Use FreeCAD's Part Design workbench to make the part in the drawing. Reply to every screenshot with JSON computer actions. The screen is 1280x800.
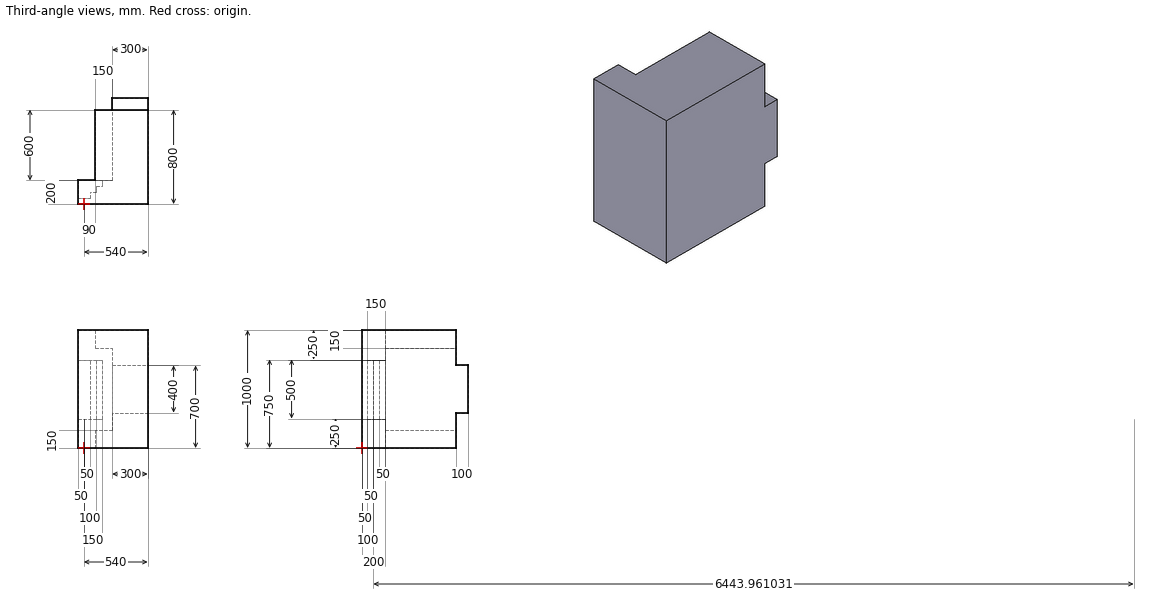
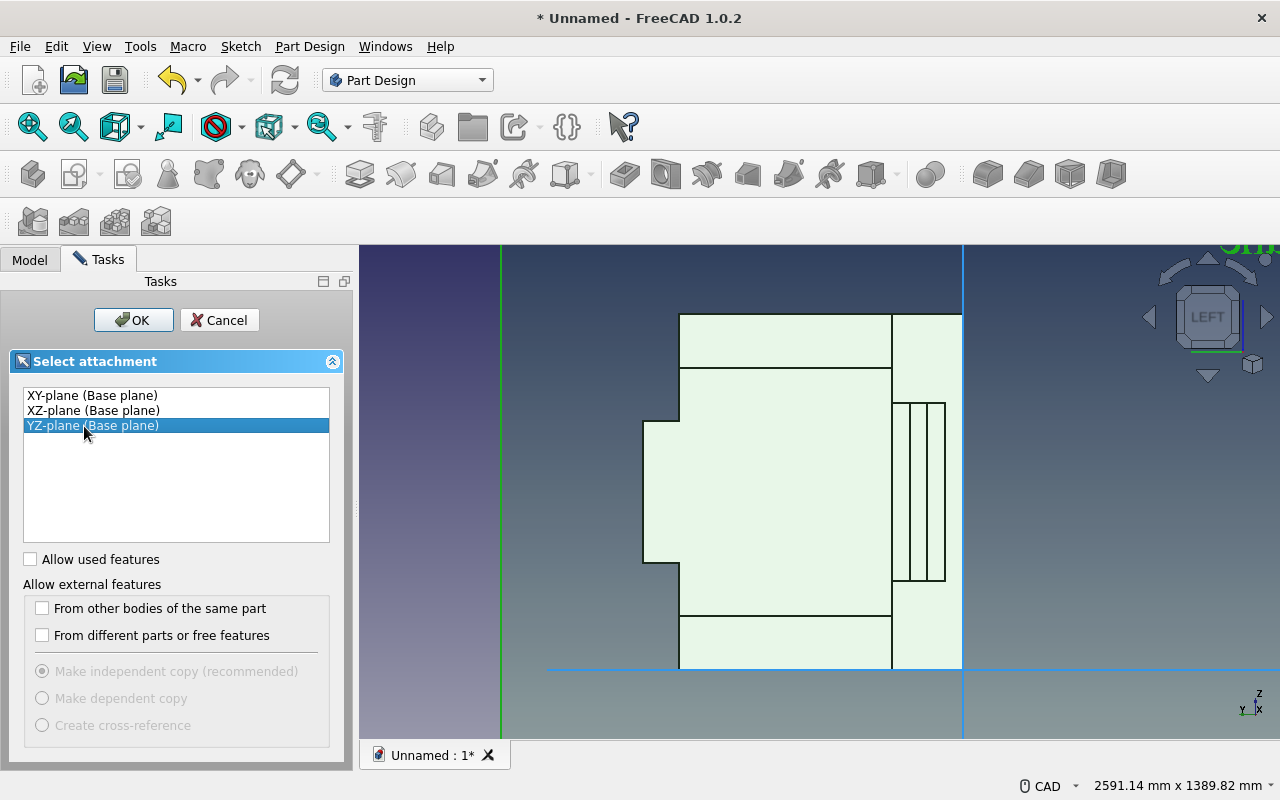
{"action": "left_click", "coordinate": [134, 320]}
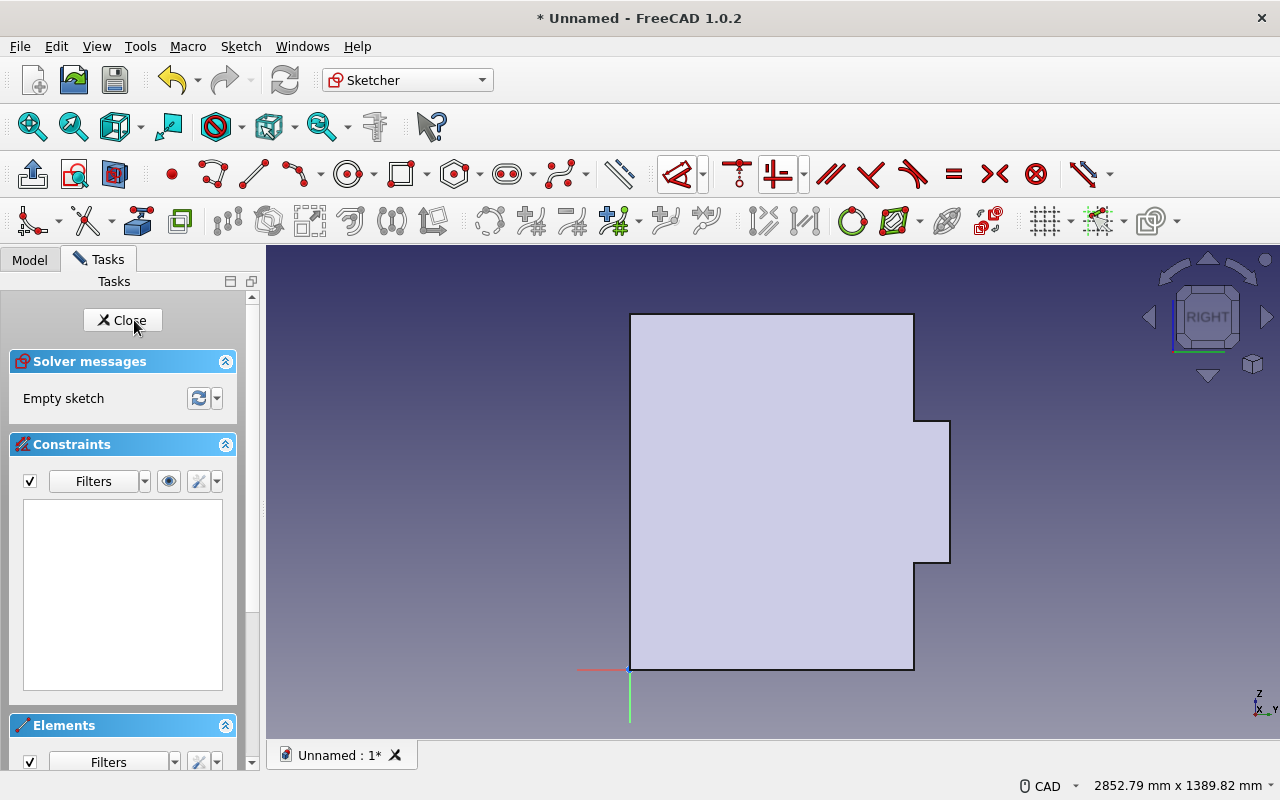
{"action": "left_click", "coordinate": [115, 174]}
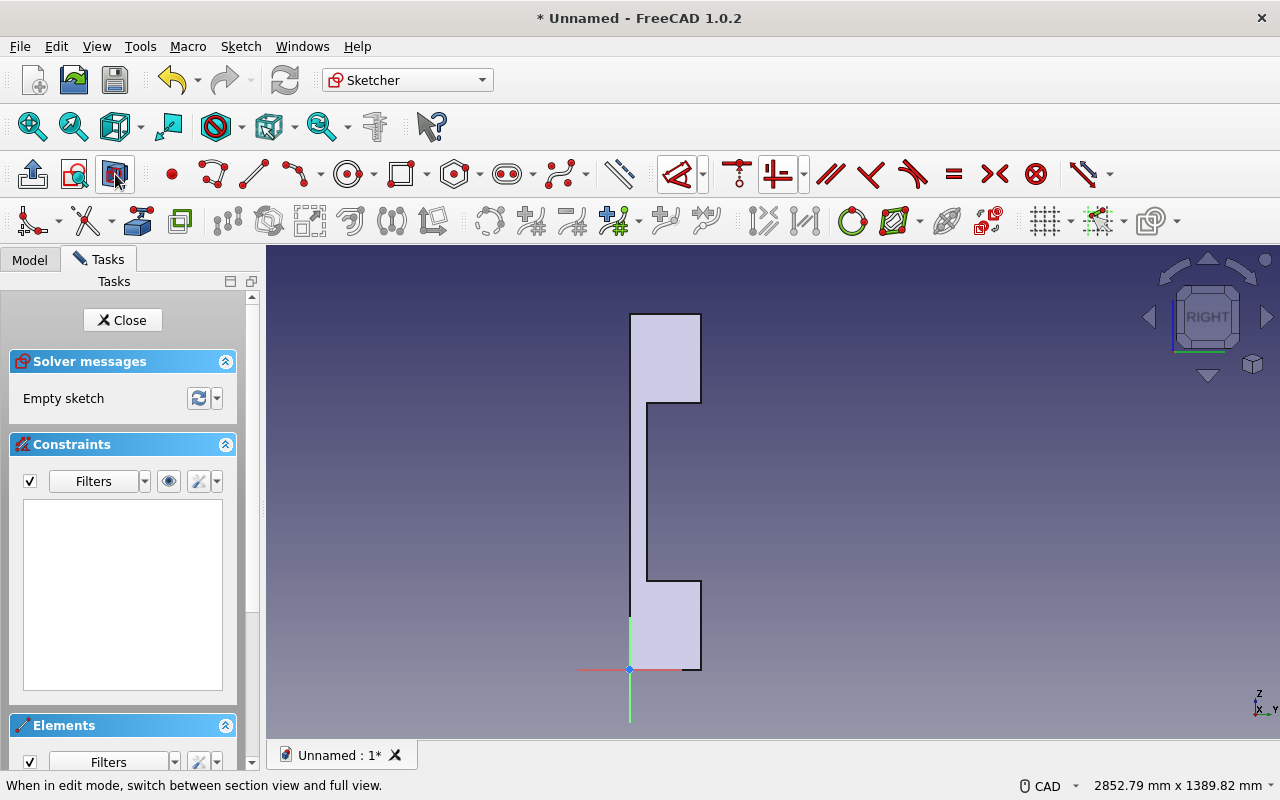
{"action": "left_click", "coordinate": [213, 174]}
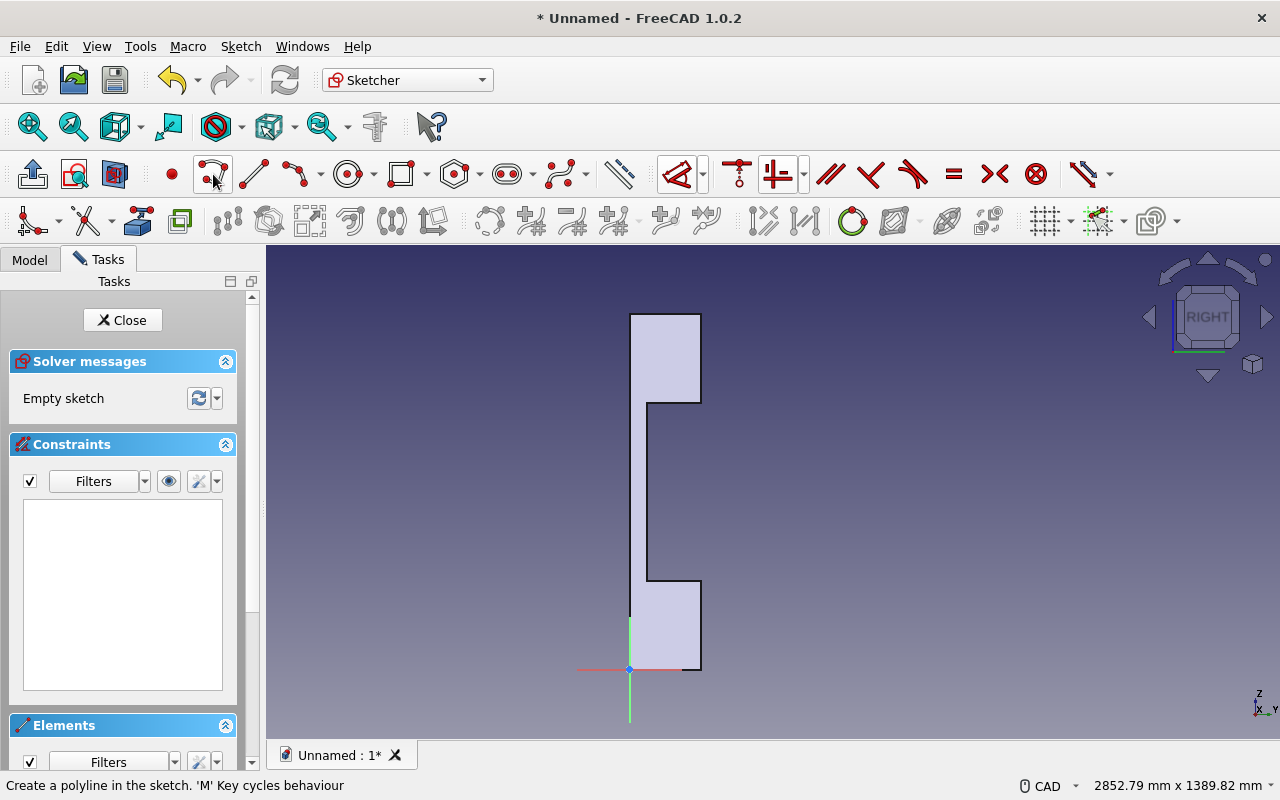
{"action": "left_click", "coordinate": [630, 670]}
{"action": "left_click", "coordinate": [639, 314]}
{"action": "left_click", "coordinate": [701, 314]}
{"action": "left_click", "coordinate": [701, 403]}
{"action": "left_click", "coordinate": [647, 403]}
{"action": "left_click", "coordinate": [647, 581]}
{"action": "left_click", "coordinate": [701, 581]}
{"action": "left_click", "coordinate": [701, 661]}
{"action": "left_click", "coordinate": [630, 670]}
{"action": "key", "text": "Escape"}
{"action": "key", "text": "Escape"}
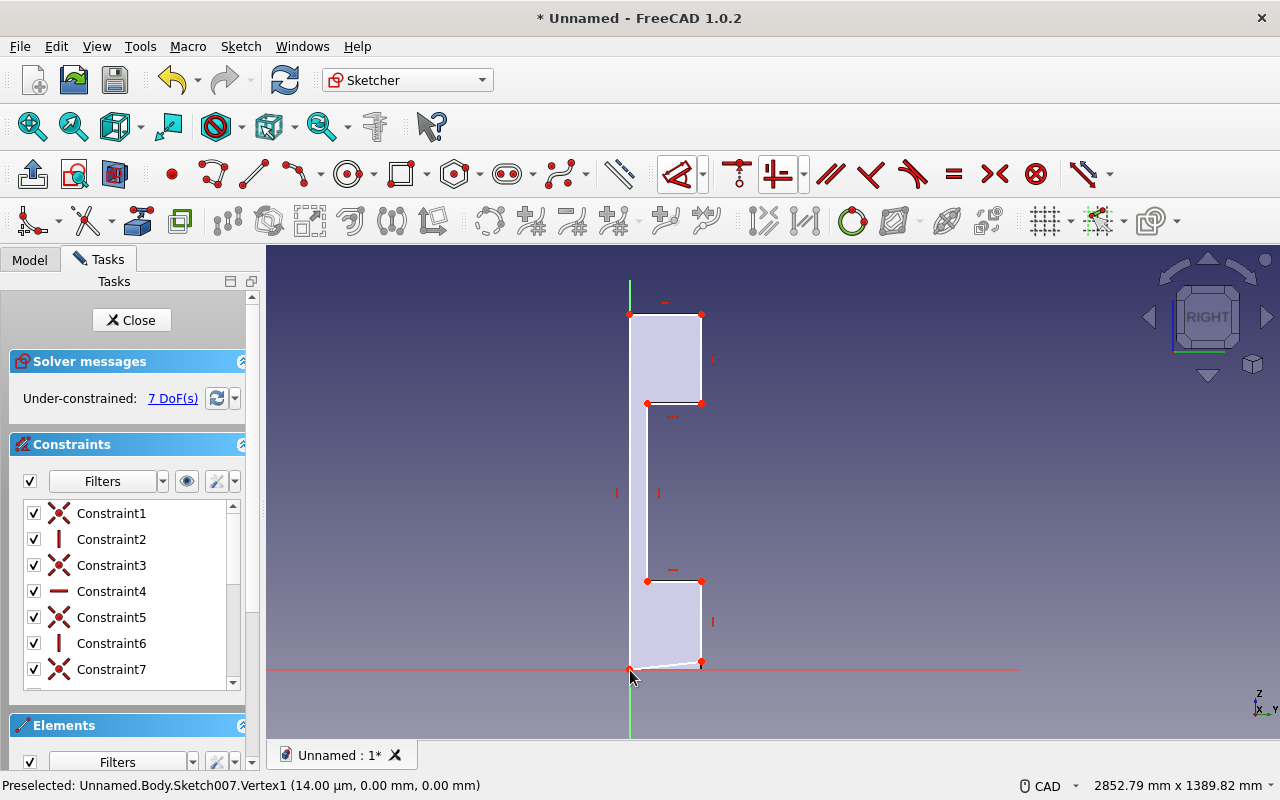
{"action": "left_click", "coordinate": [651, 667]}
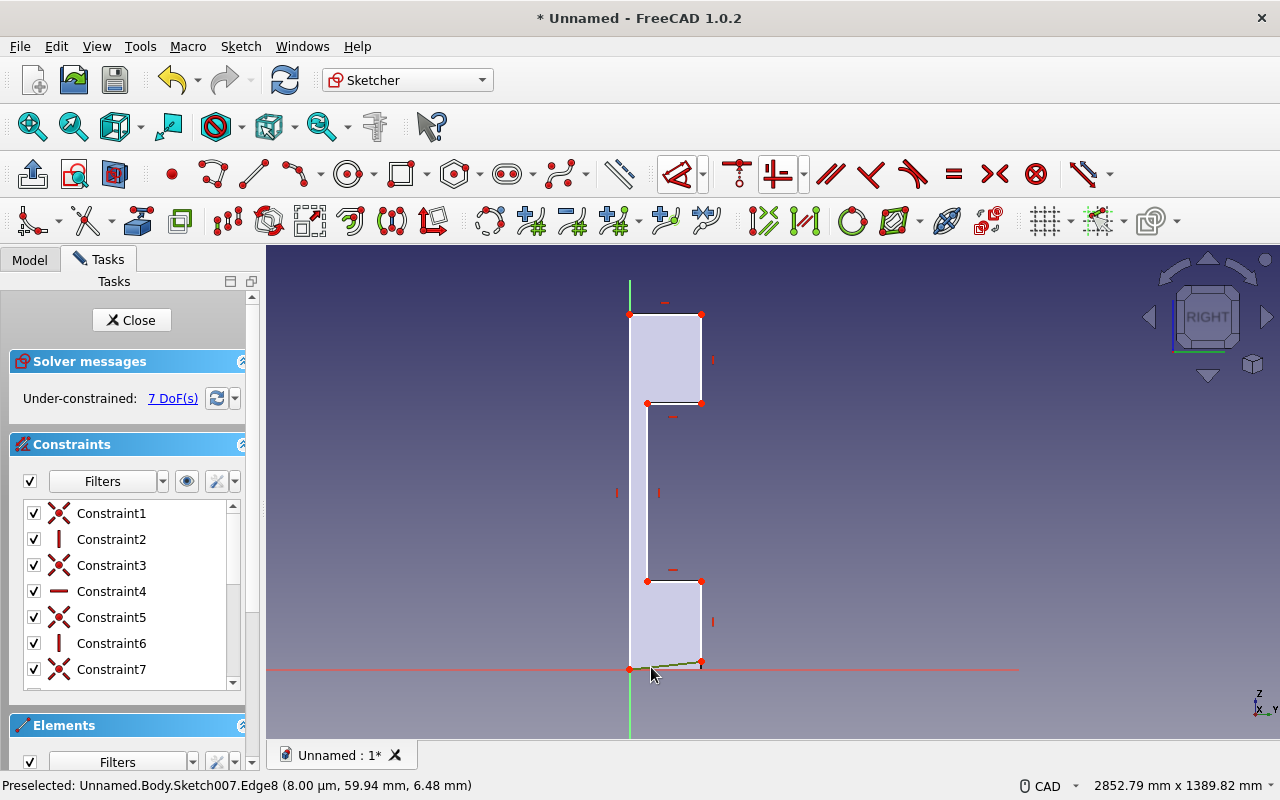
{"action": "key", "text": "h"}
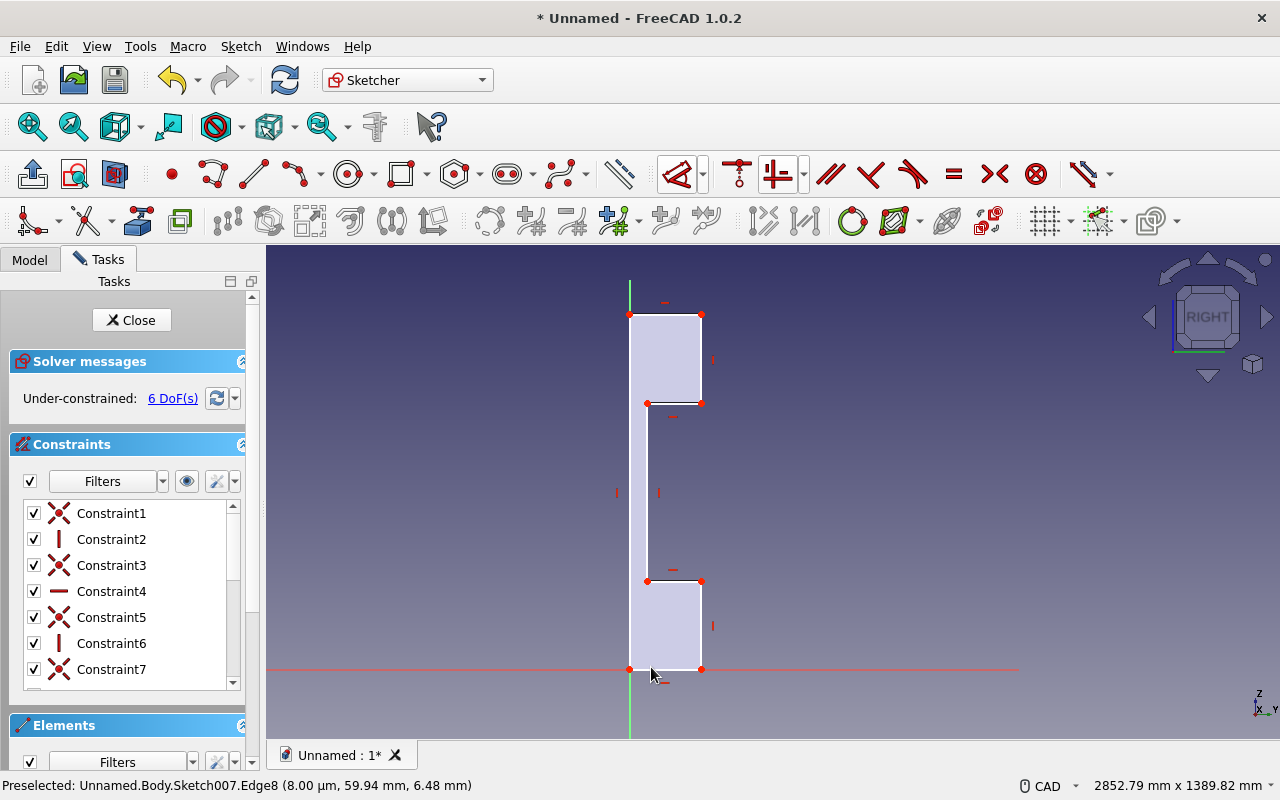
{"action": "left_click", "coordinate": [651, 315]}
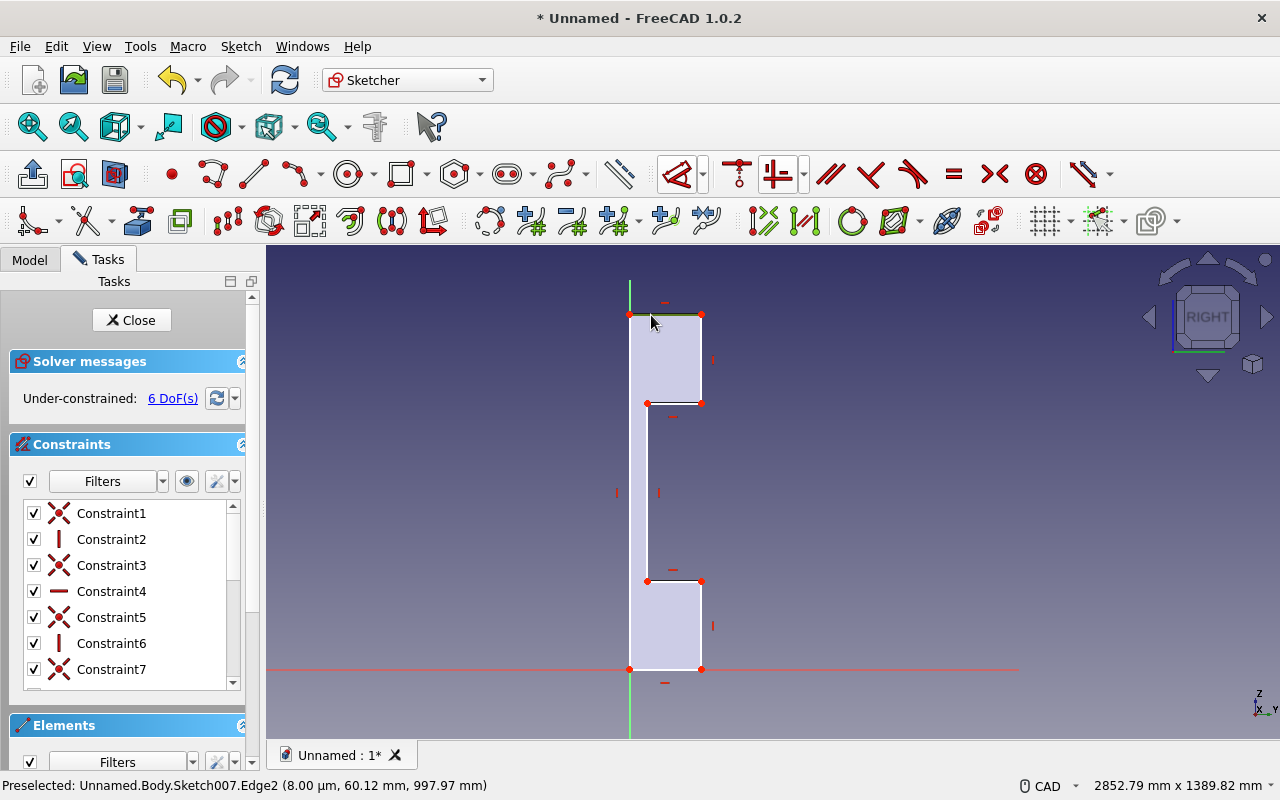
{"action": "left_click", "coordinate": [702, 174]}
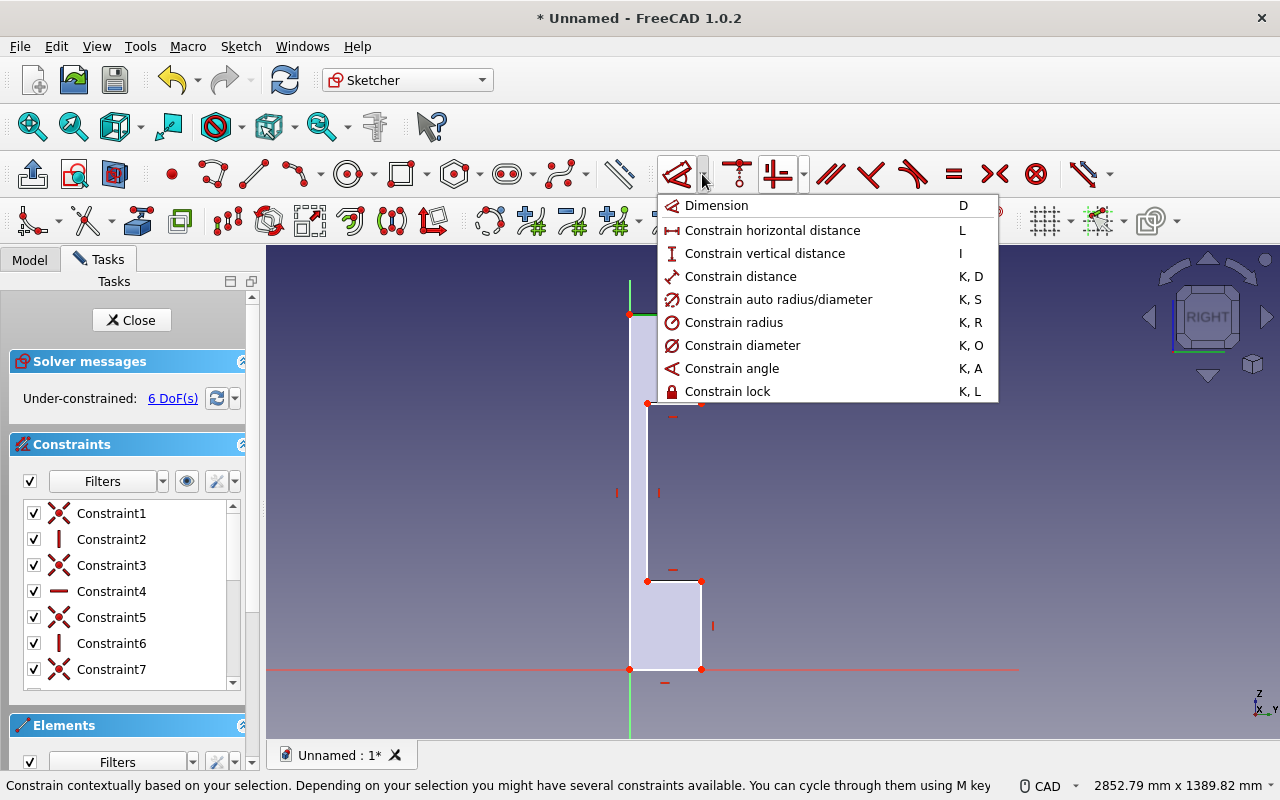
{"action": "left_click", "coordinate": [828, 230]}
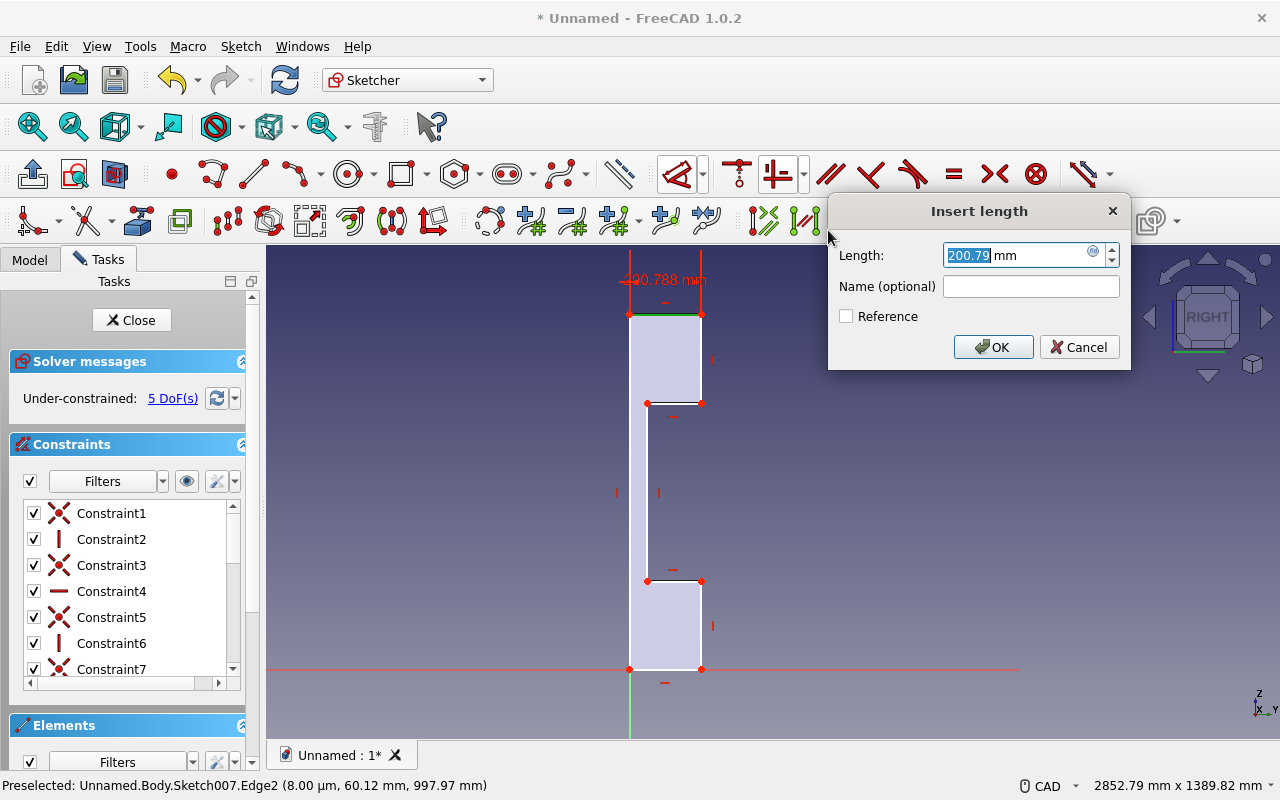
{"action": "type", "text": "200"}
{"action": "key", "text": "Return"}